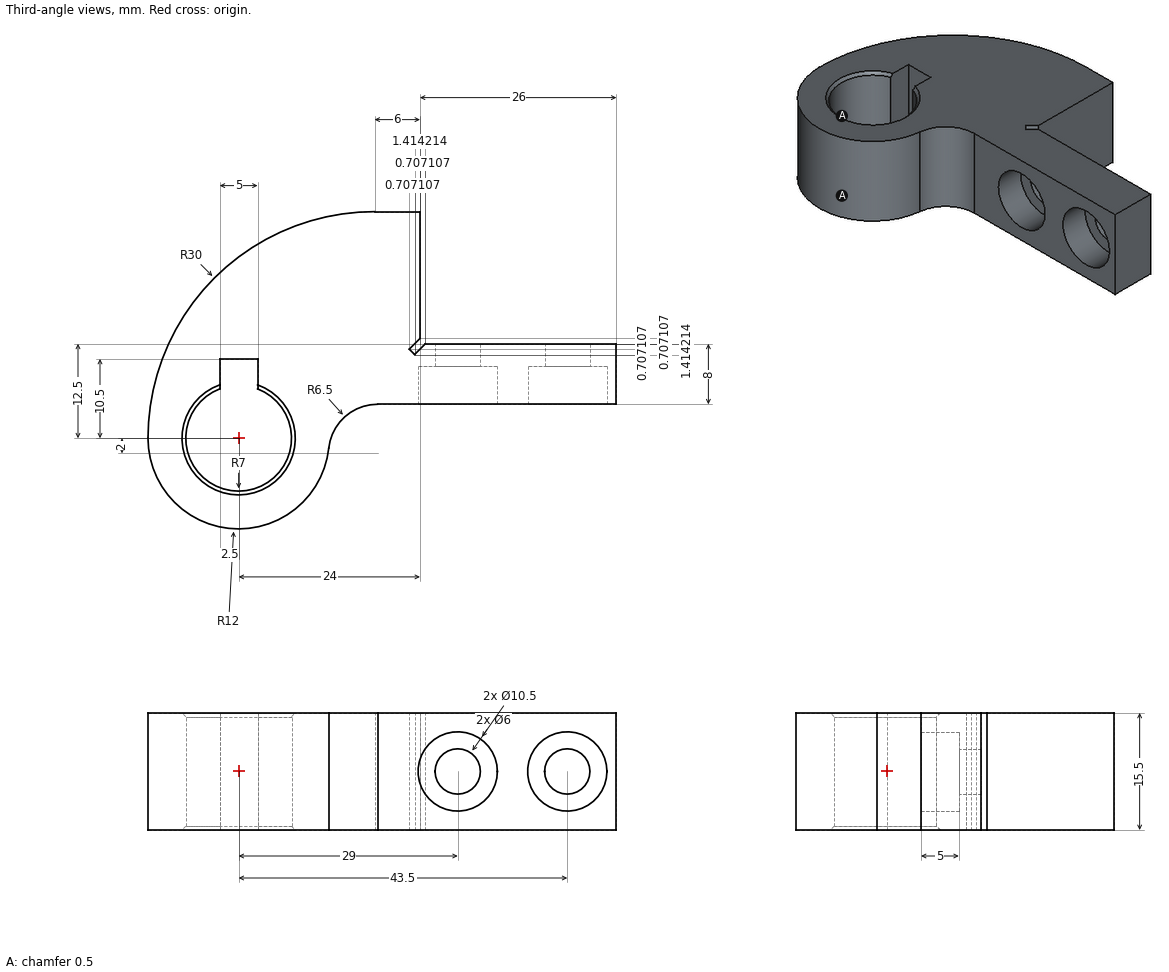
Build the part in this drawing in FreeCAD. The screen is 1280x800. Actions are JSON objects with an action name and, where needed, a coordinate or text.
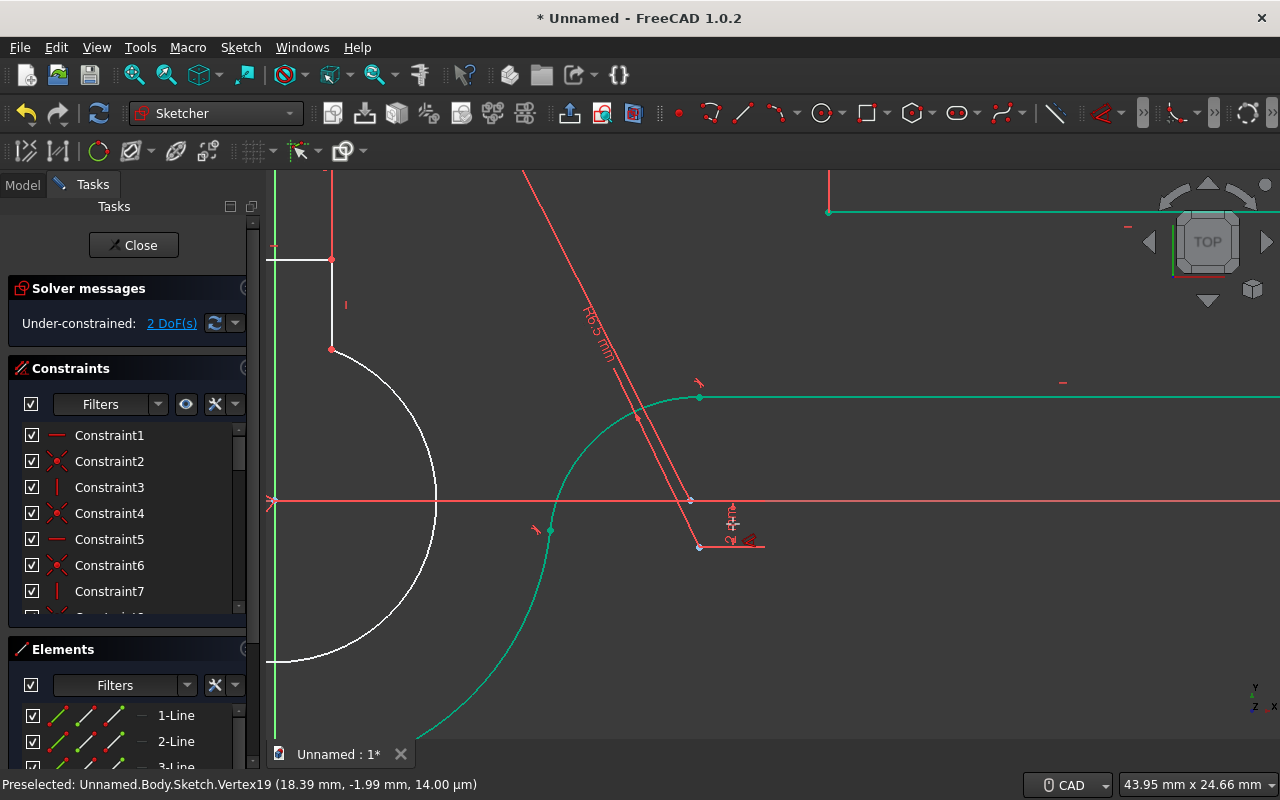
{"action": "scroll", "coordinate": [699, 548], "scroll_direction": "down", "scroll_amount": 5}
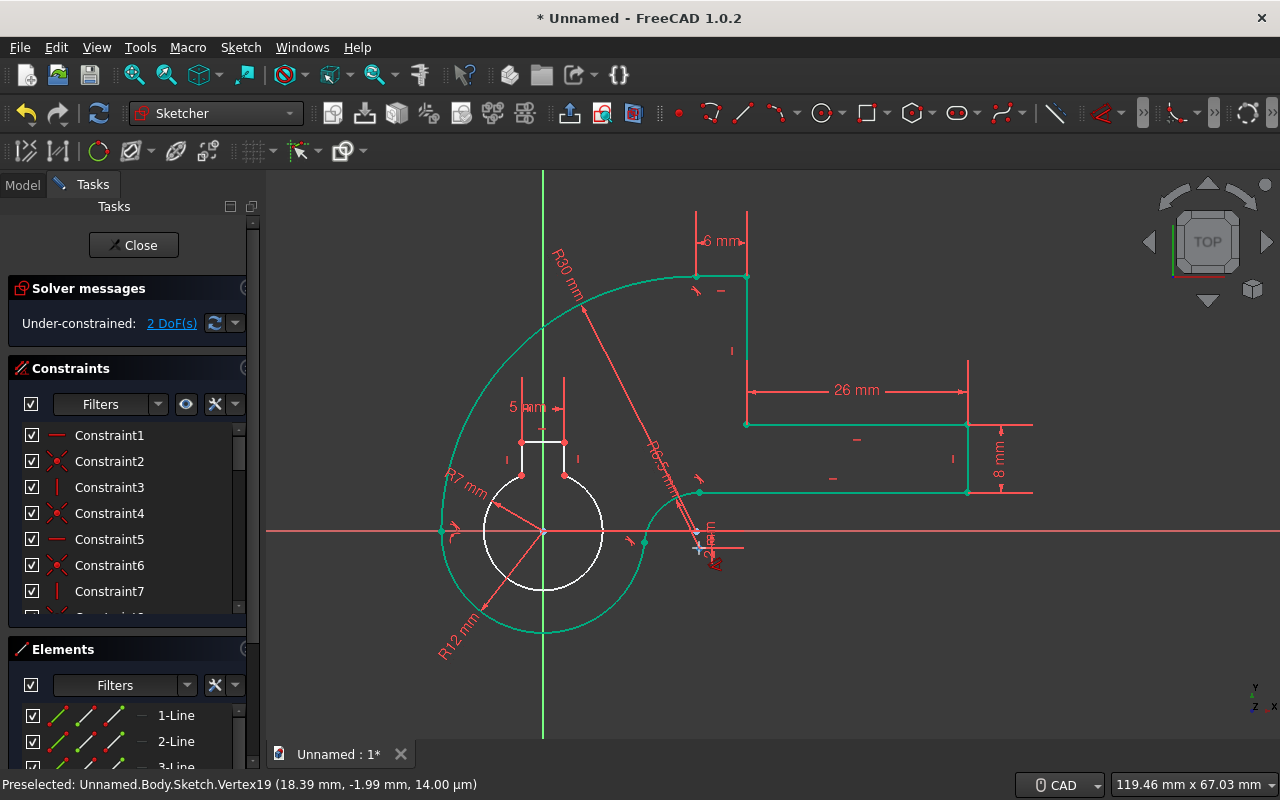
{"action": "scroll", "coordinate": [522, 476], "scroll_direction": "up", "scroll_amount": 4}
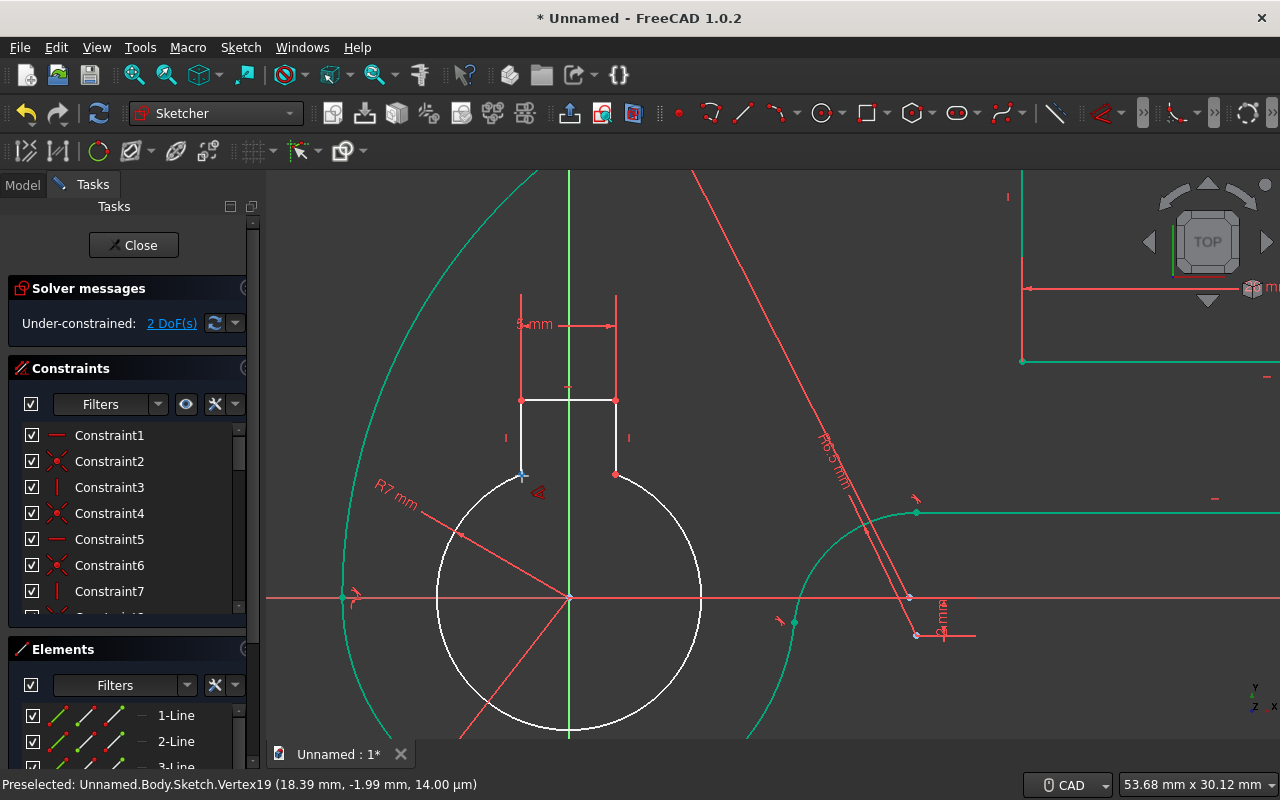
{"action": "left_click", "coordinate": [521, 475]}
{"action": "left_click", "coordinate": [545, 632]}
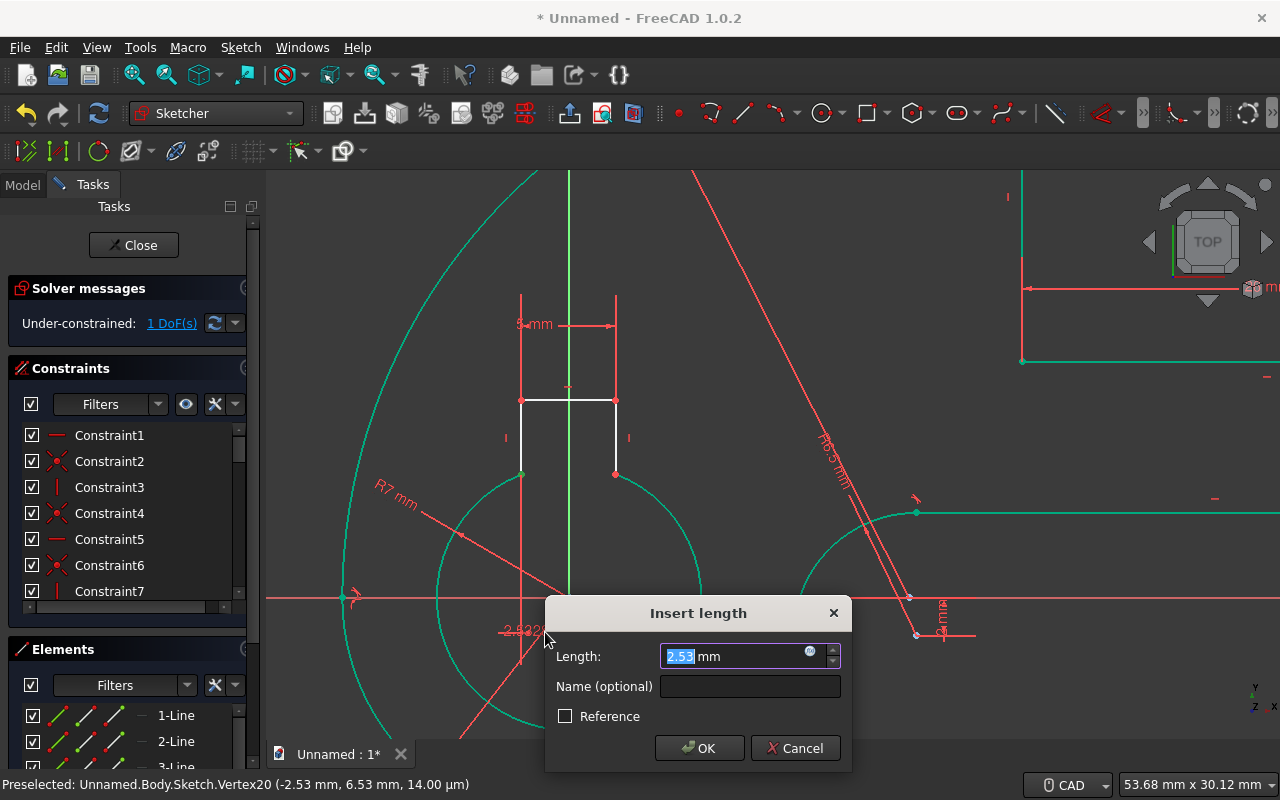
{"action": "type", "text": "2.5"}
{"action": "key", "text": "Return"}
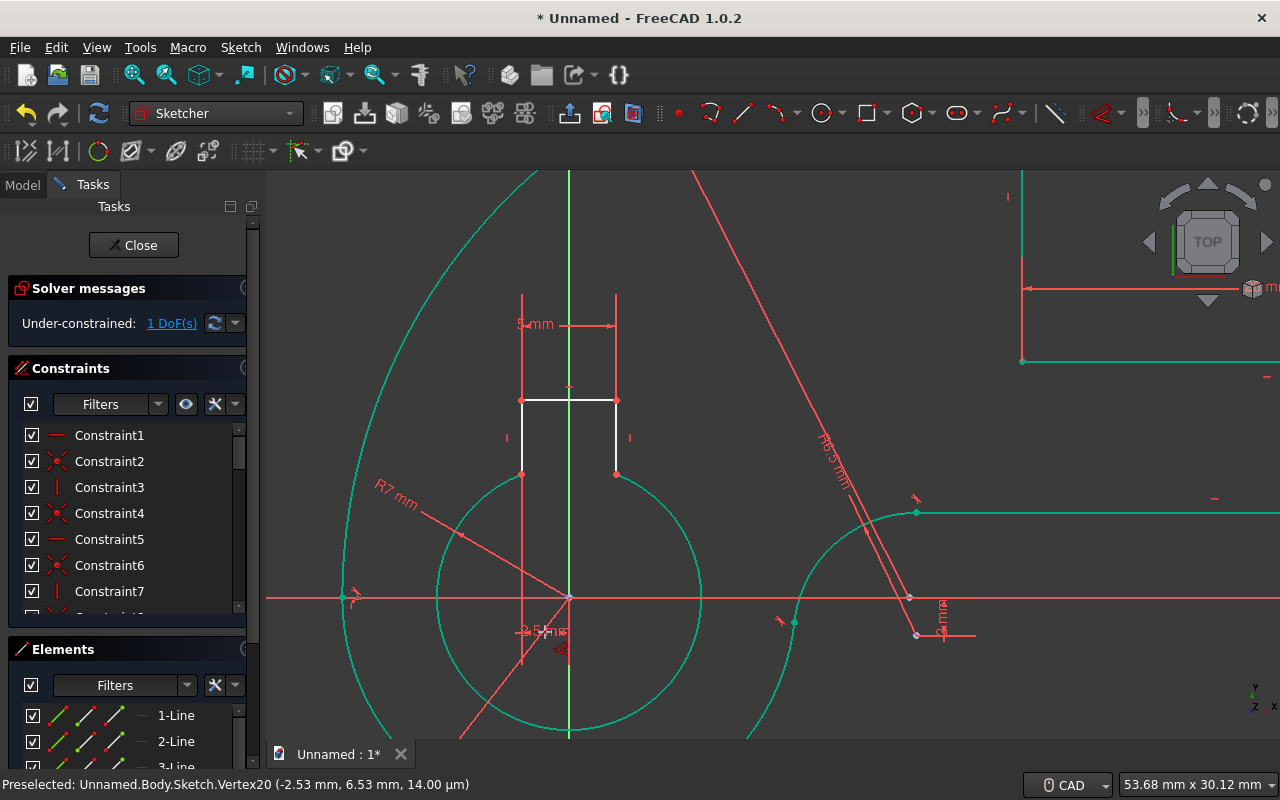
{"action": "left_click", "coordinate": [522, 400]}
{"action": "left_click", "coordinate": [488, 454]}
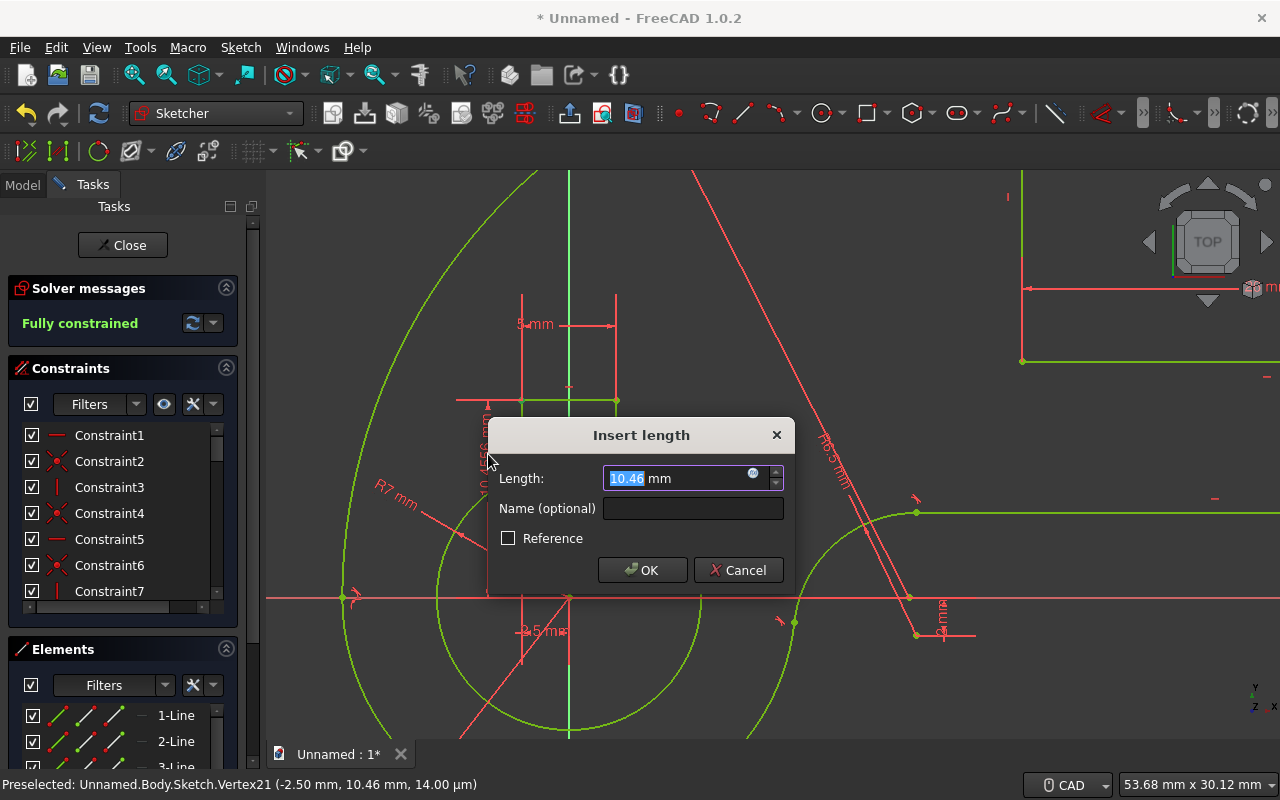
{"action": "type", "text": "10.5"}
{"action": "key", "text": "Return"}
{"action": "key", "text": "Escape"}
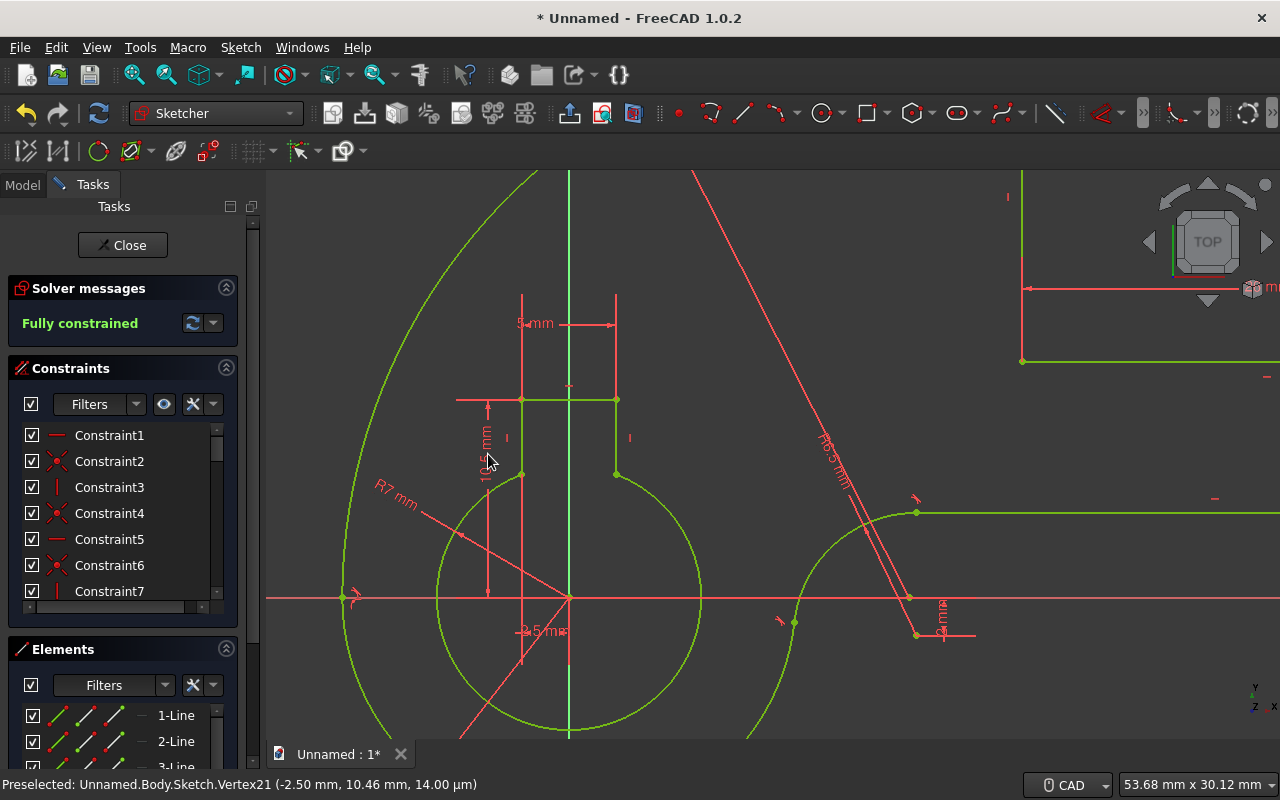
{"action": "left_click", "coordinate": [123, 245]}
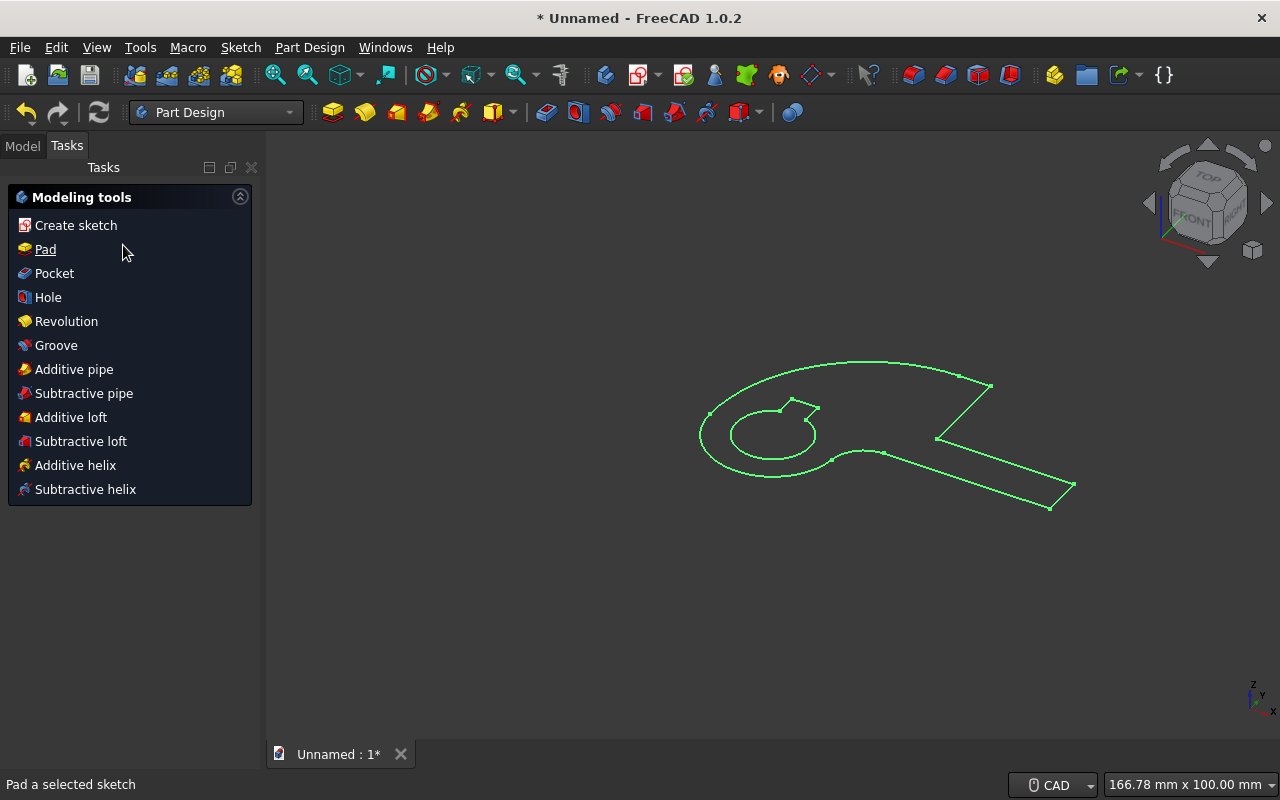
{"action": "left_click", "coordinate": [334, 112]}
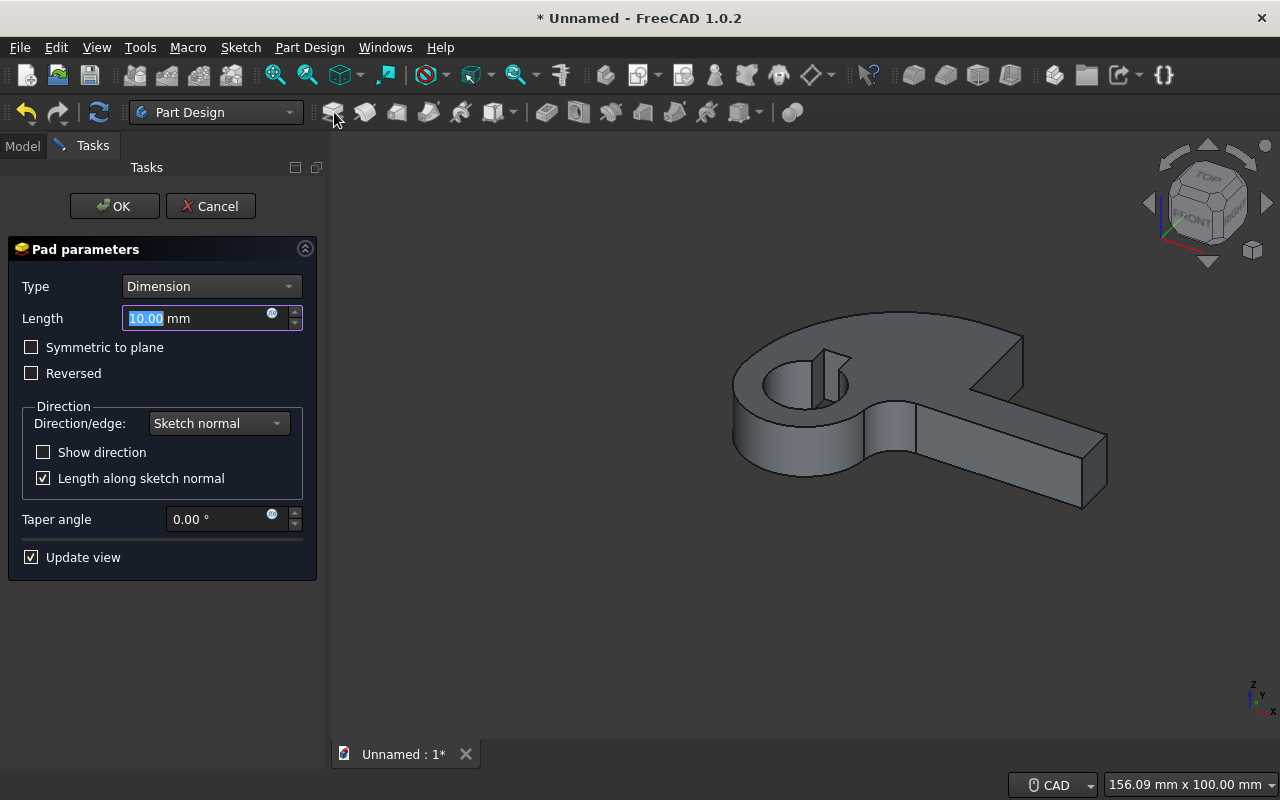
{"action": "type", "text": "15.5"}
{"action": "key", "text": "Tab"}